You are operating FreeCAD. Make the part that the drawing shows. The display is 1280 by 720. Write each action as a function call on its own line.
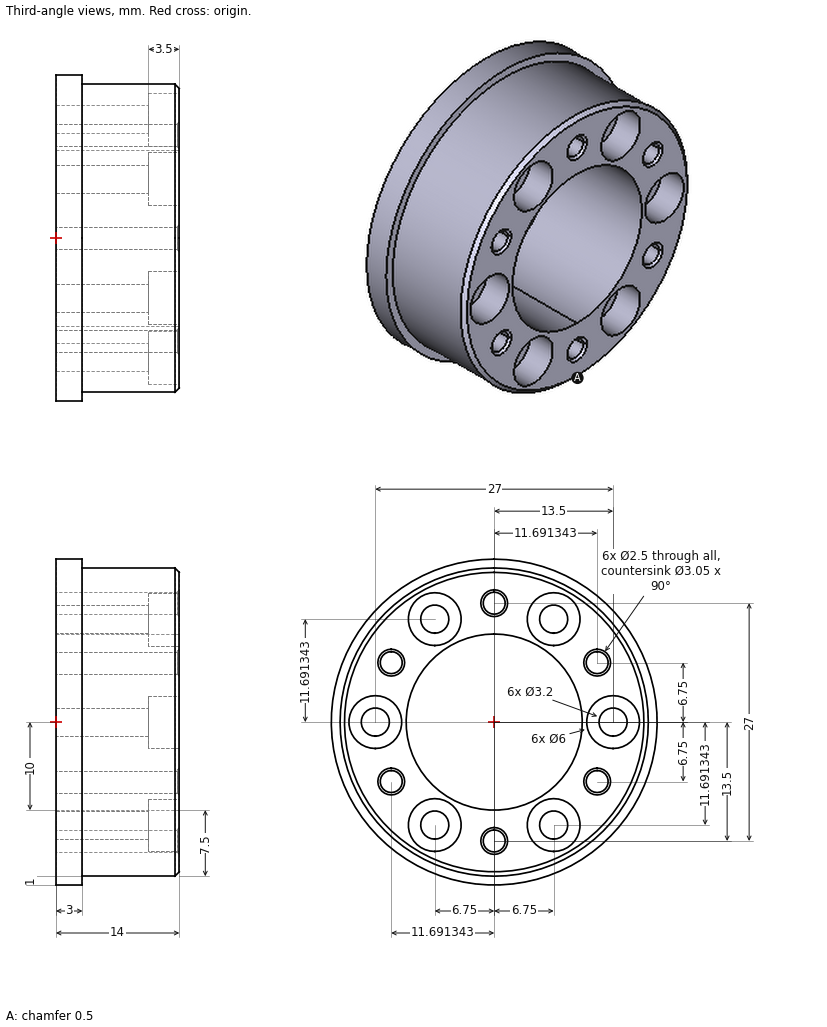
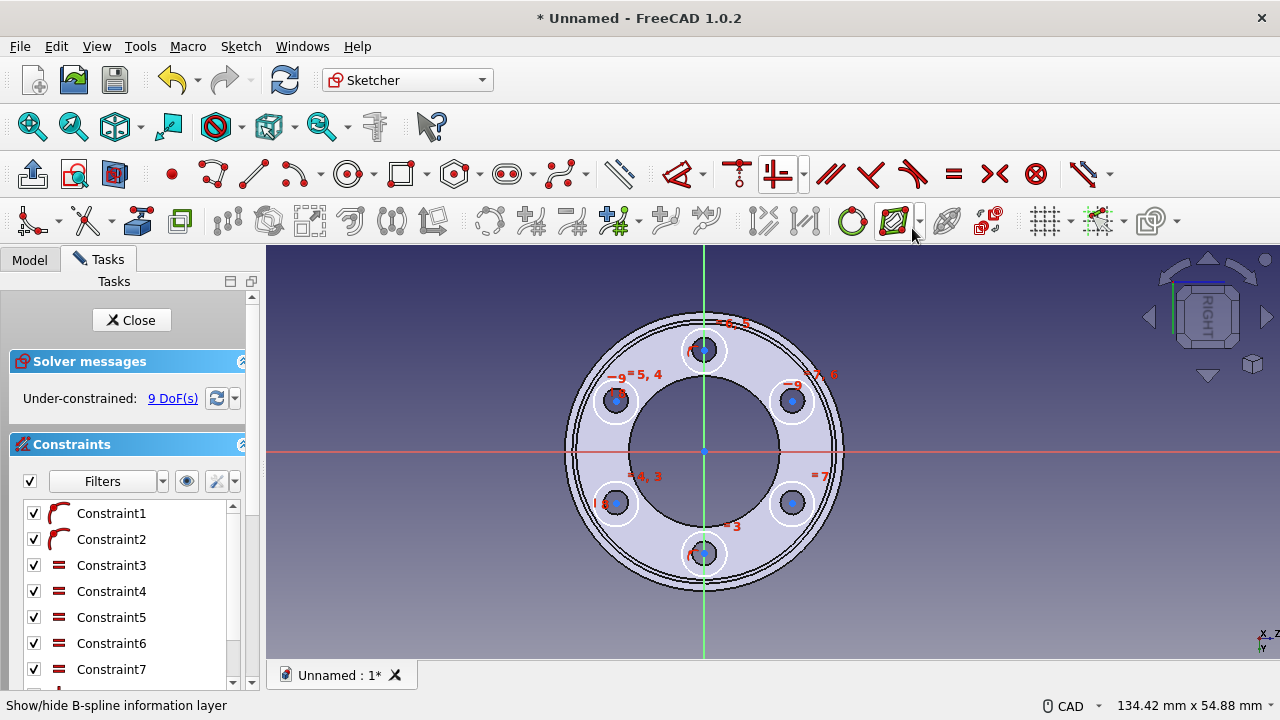
click(792, 402)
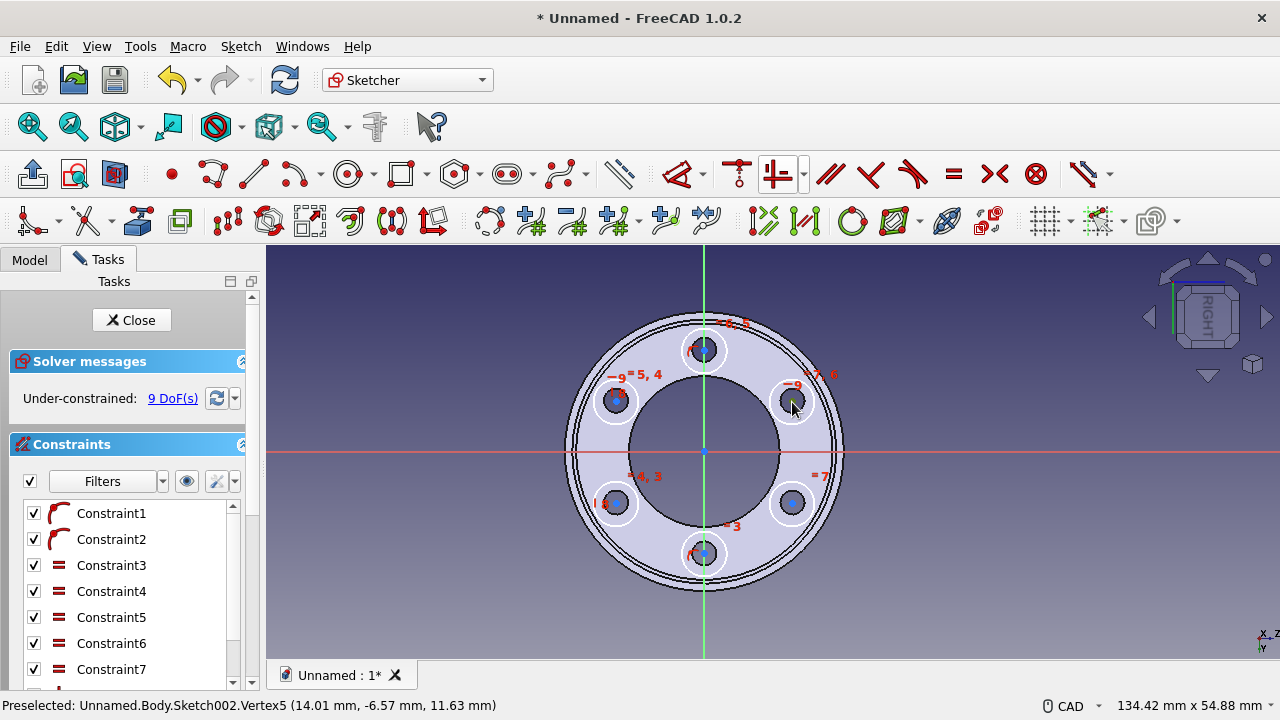
click(792, 504)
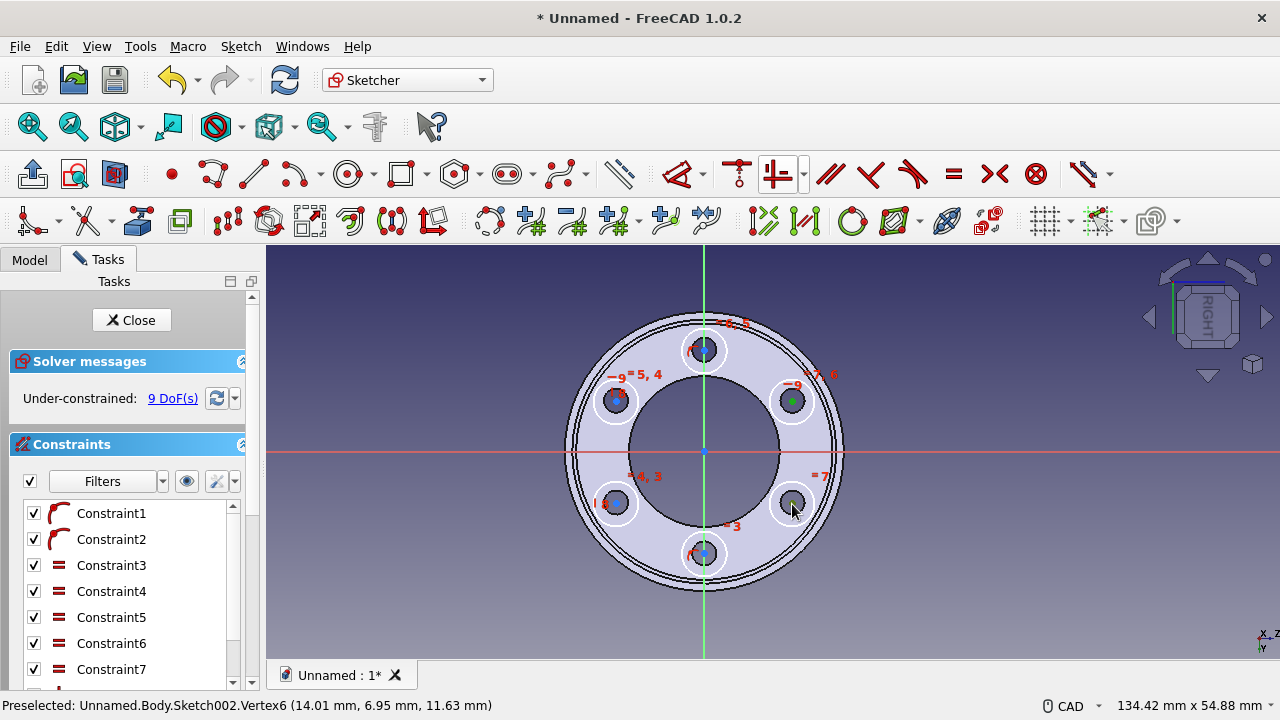
click(804, 174)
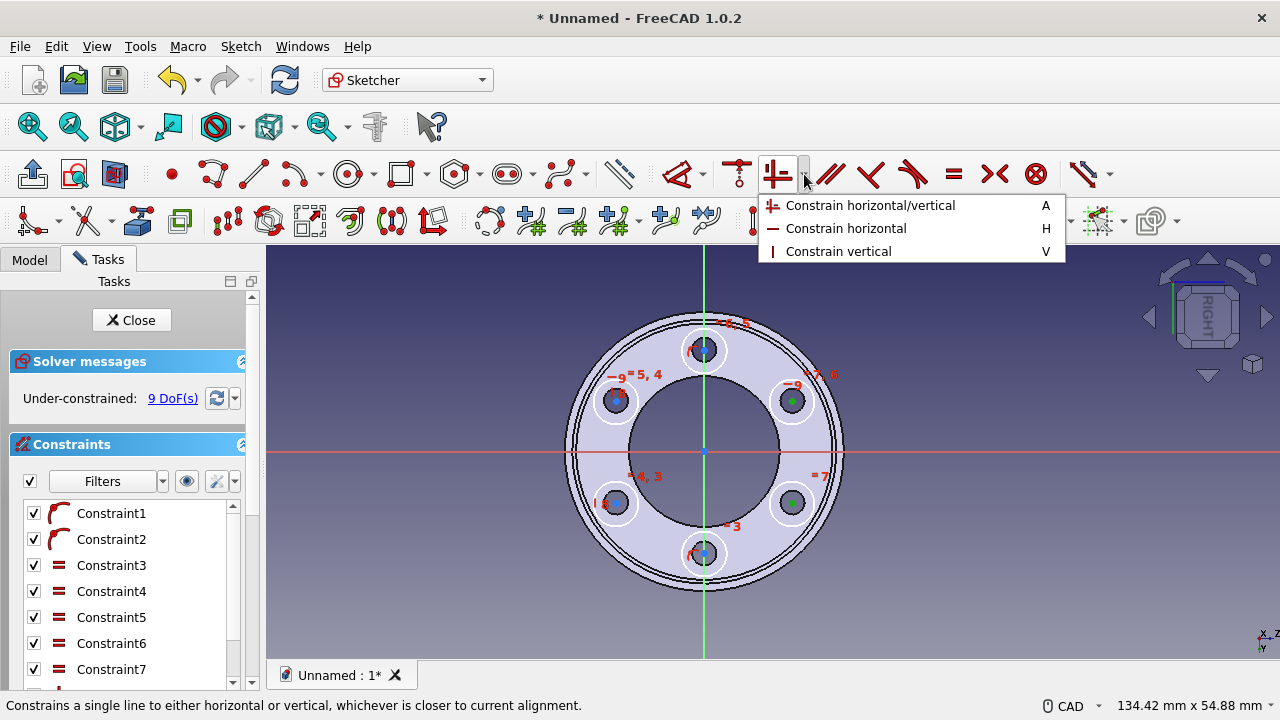
click(912, 252)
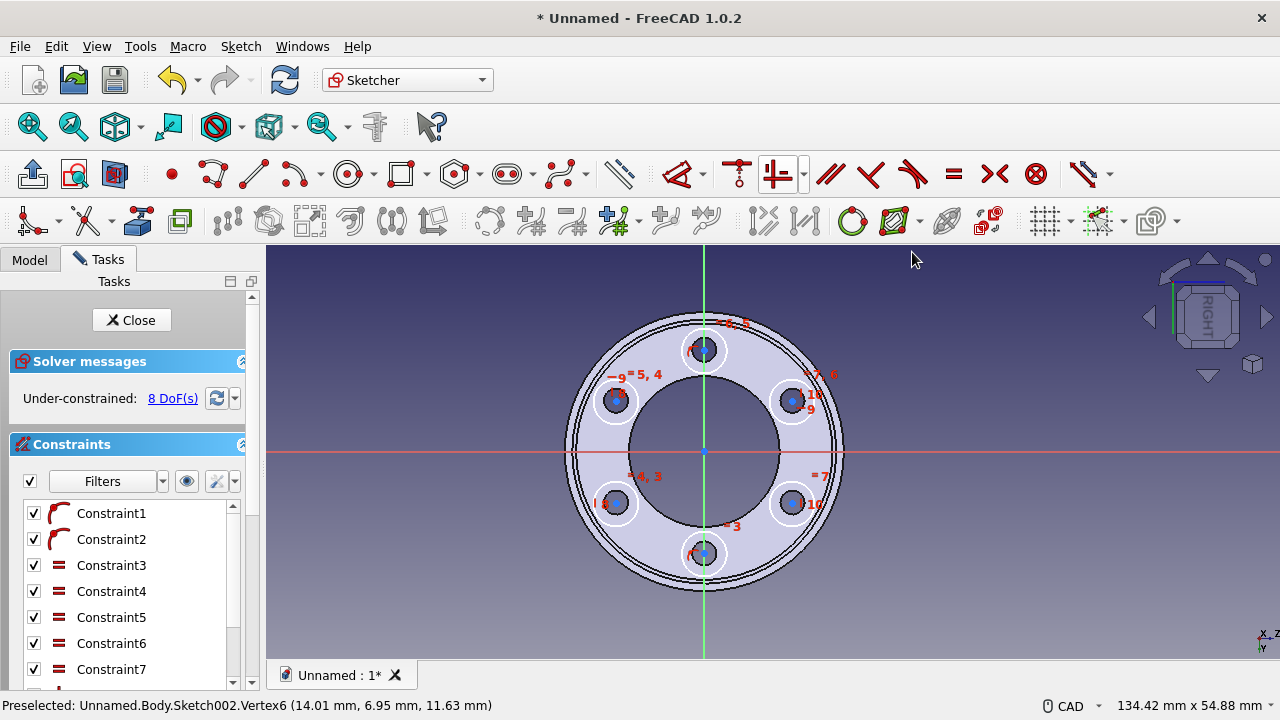
click(616, 504)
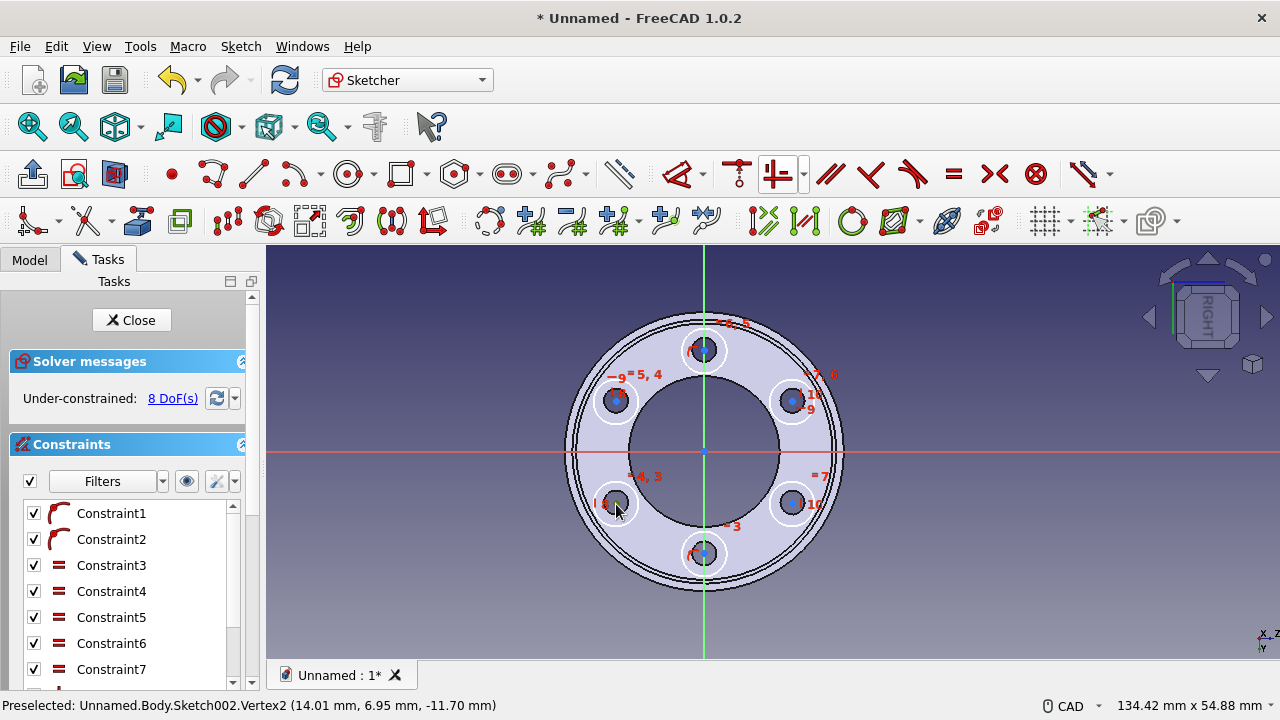
click(792, 504)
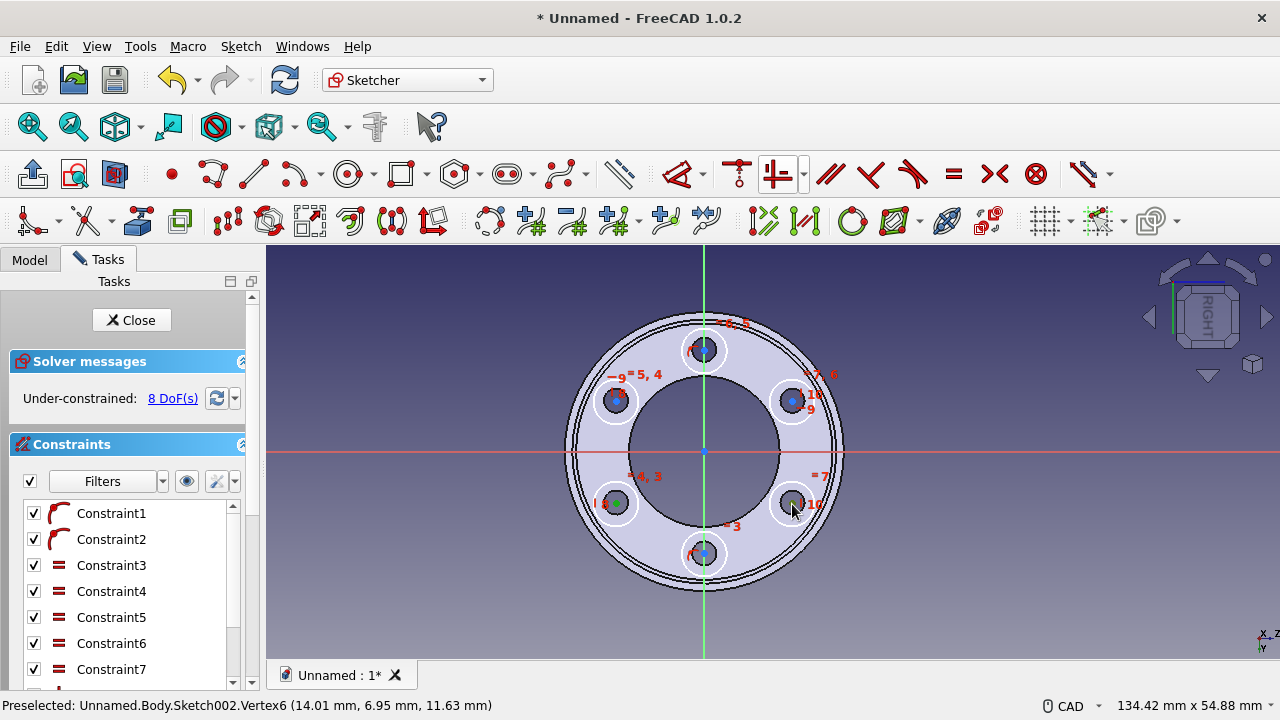
click(804, 174)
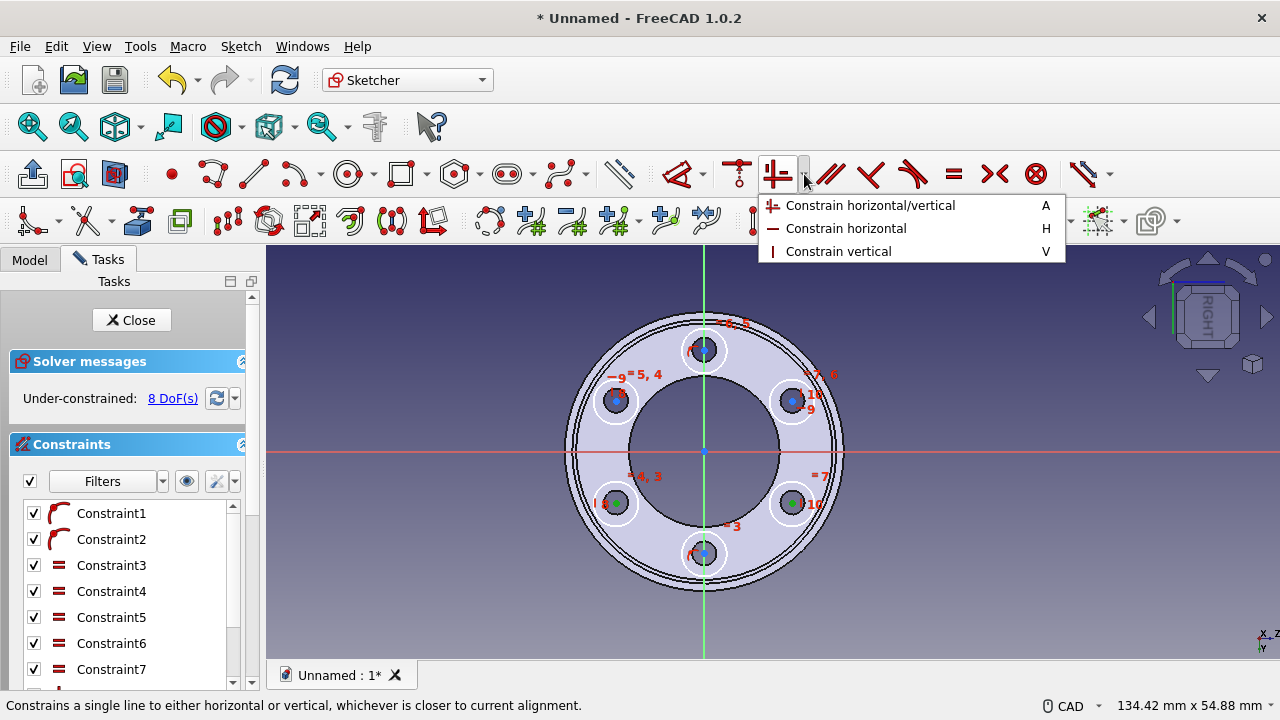
click(912, 228)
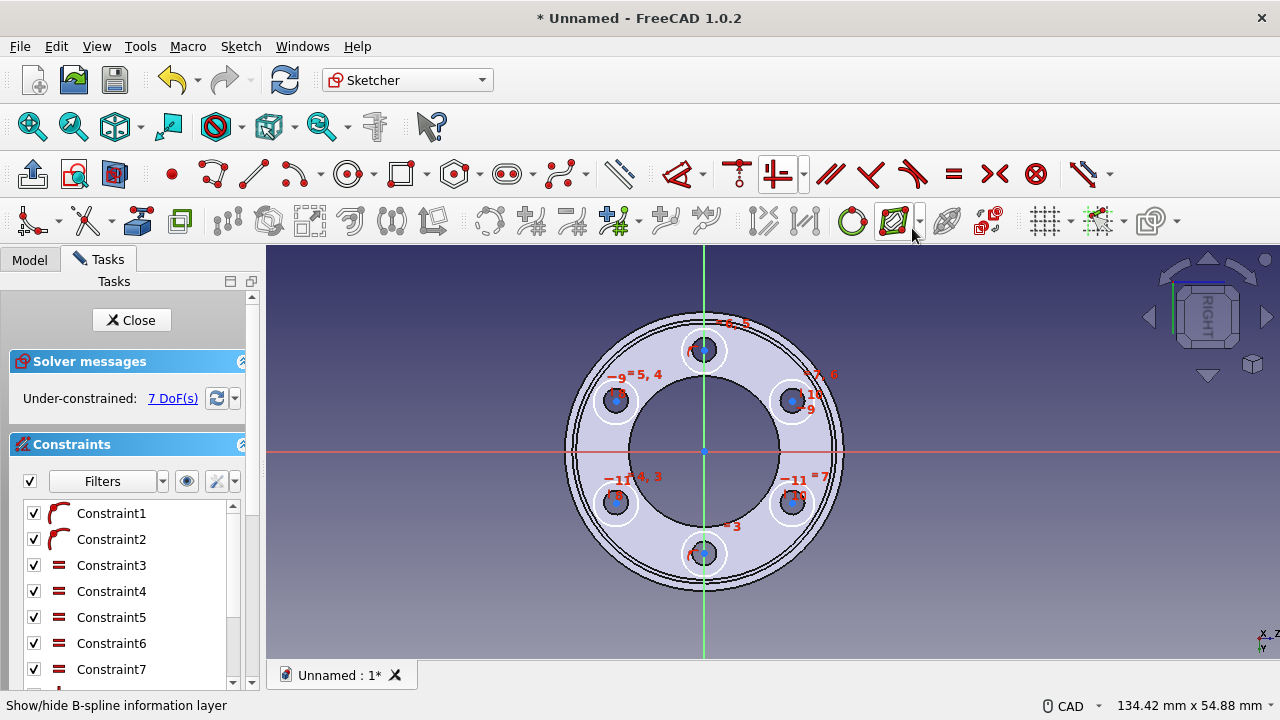
click(676, 174)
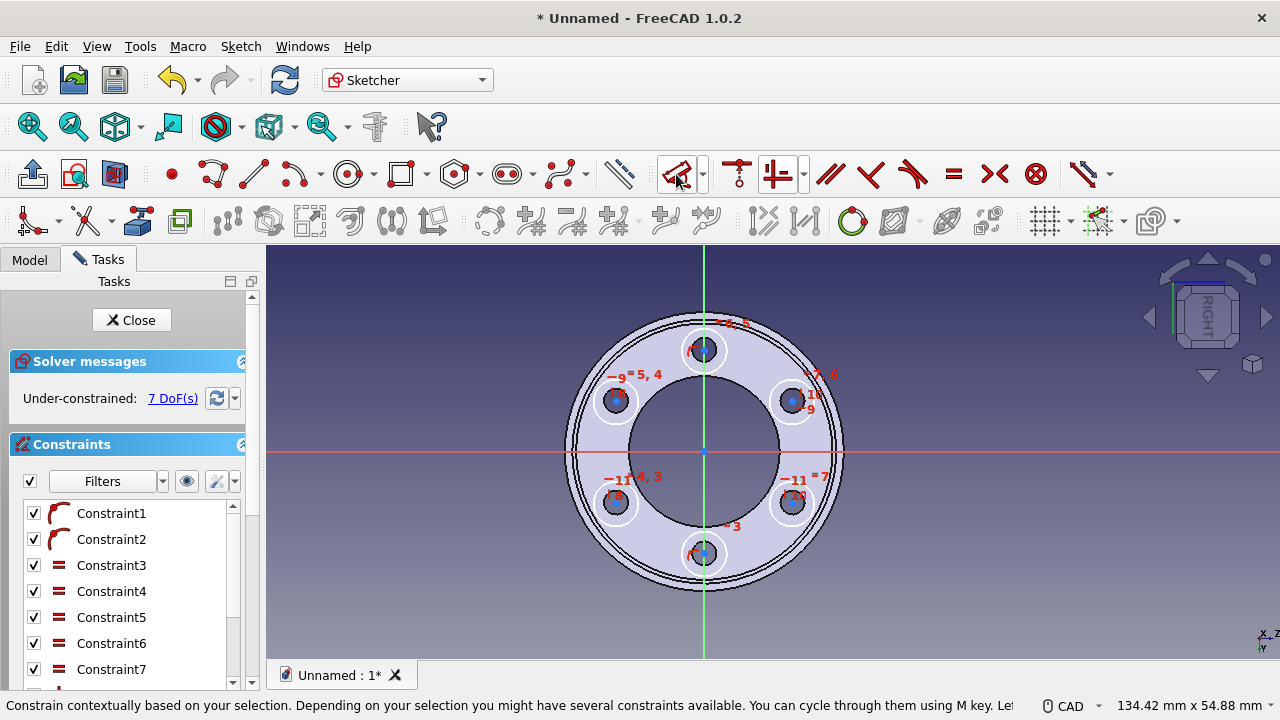
click(720, 538)
click(742, 515)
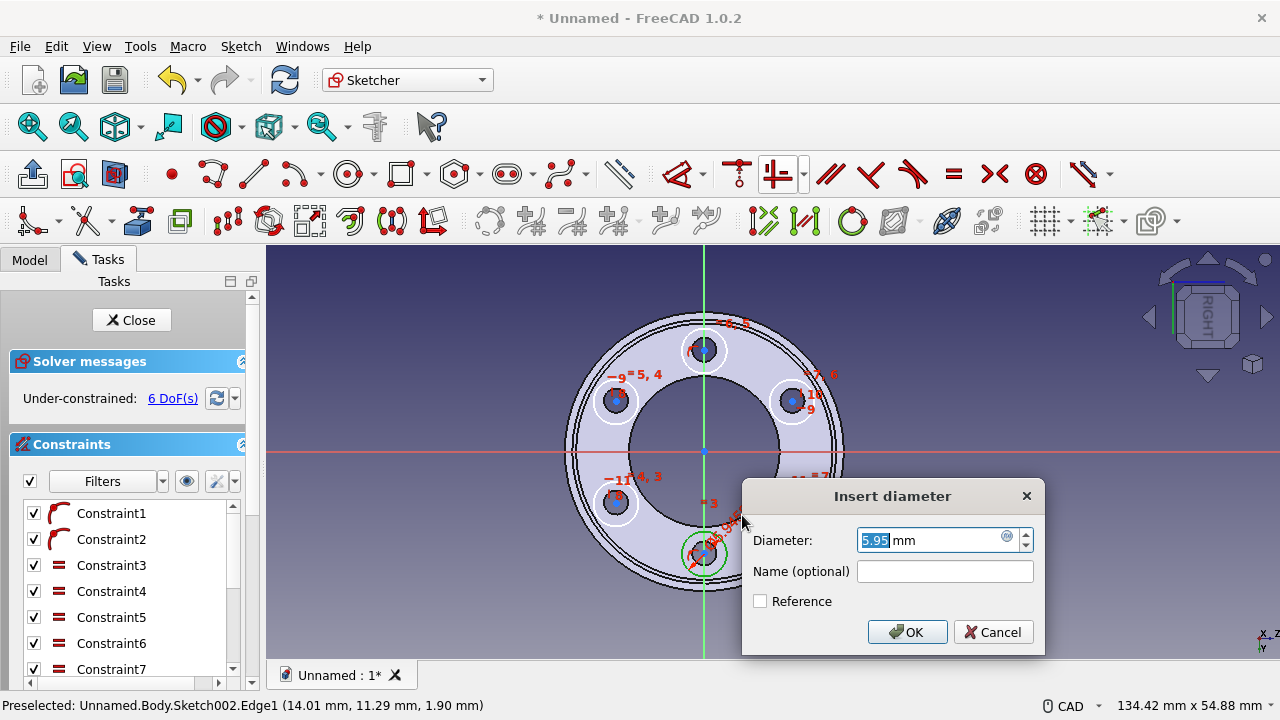
text(6)
key(Return)